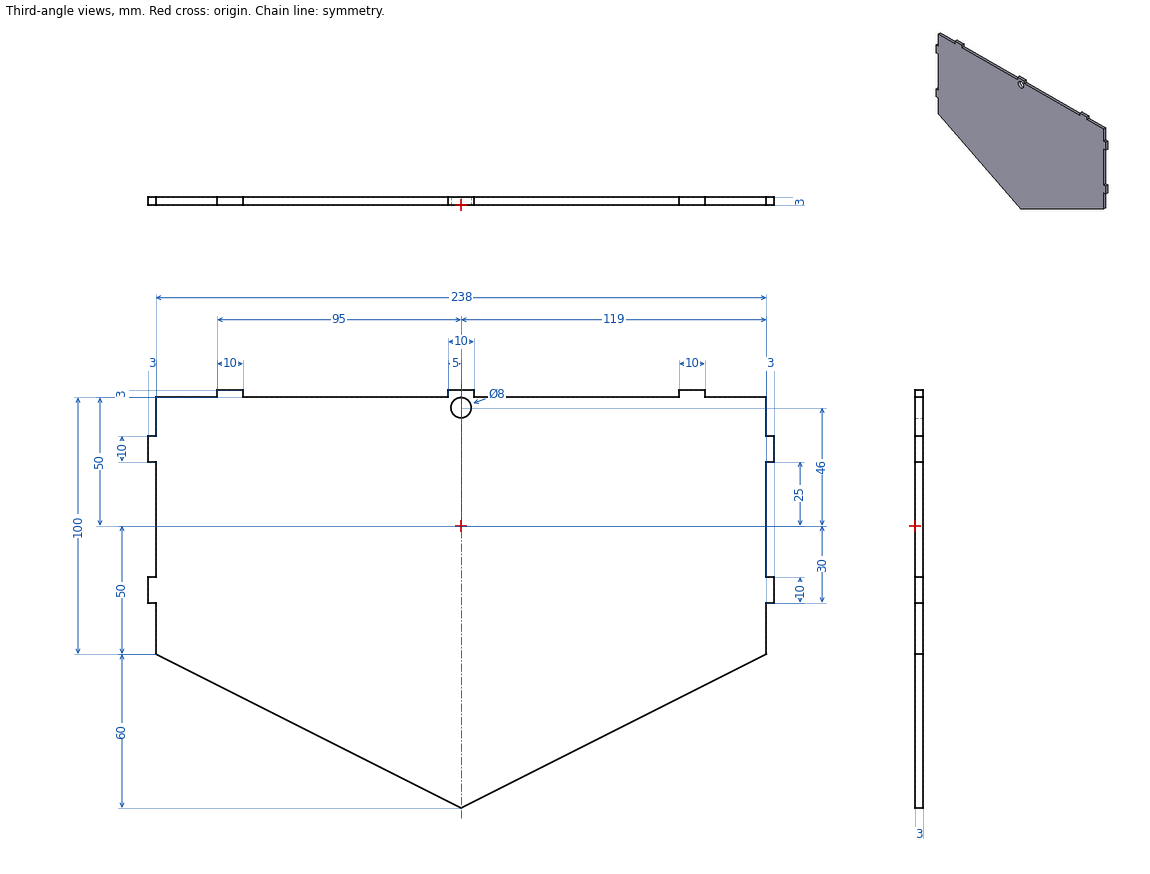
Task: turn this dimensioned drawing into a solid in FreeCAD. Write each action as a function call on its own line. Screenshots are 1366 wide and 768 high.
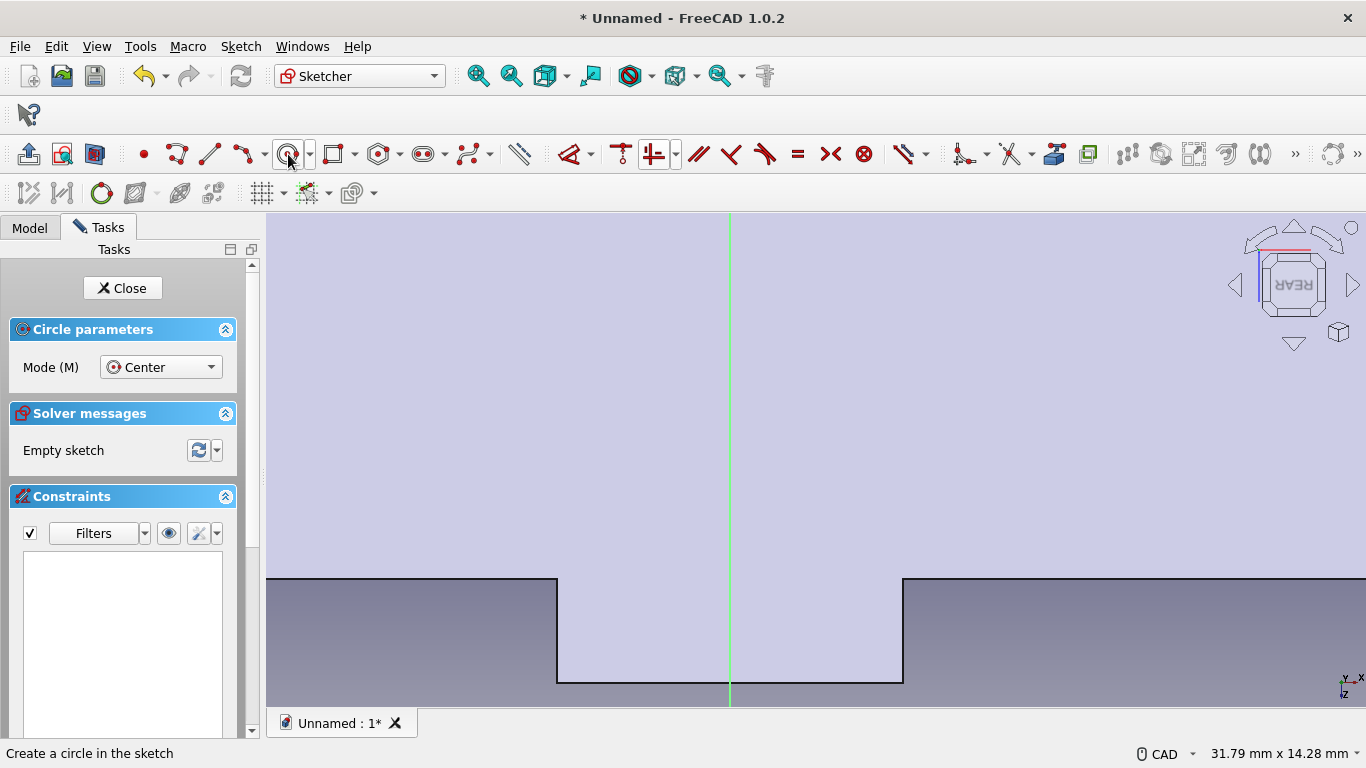
click(730, 441)
move(828, 343)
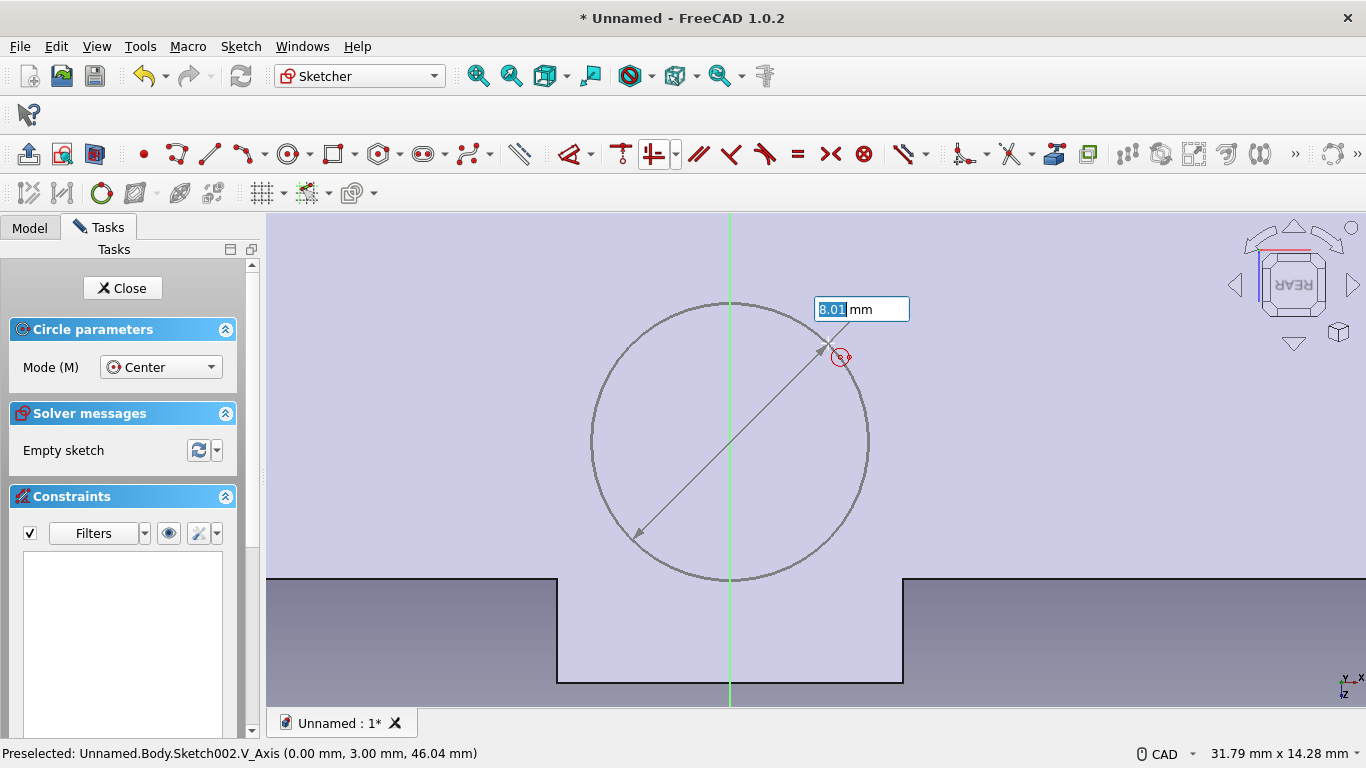
text(8)
key(Return)
key(Escape)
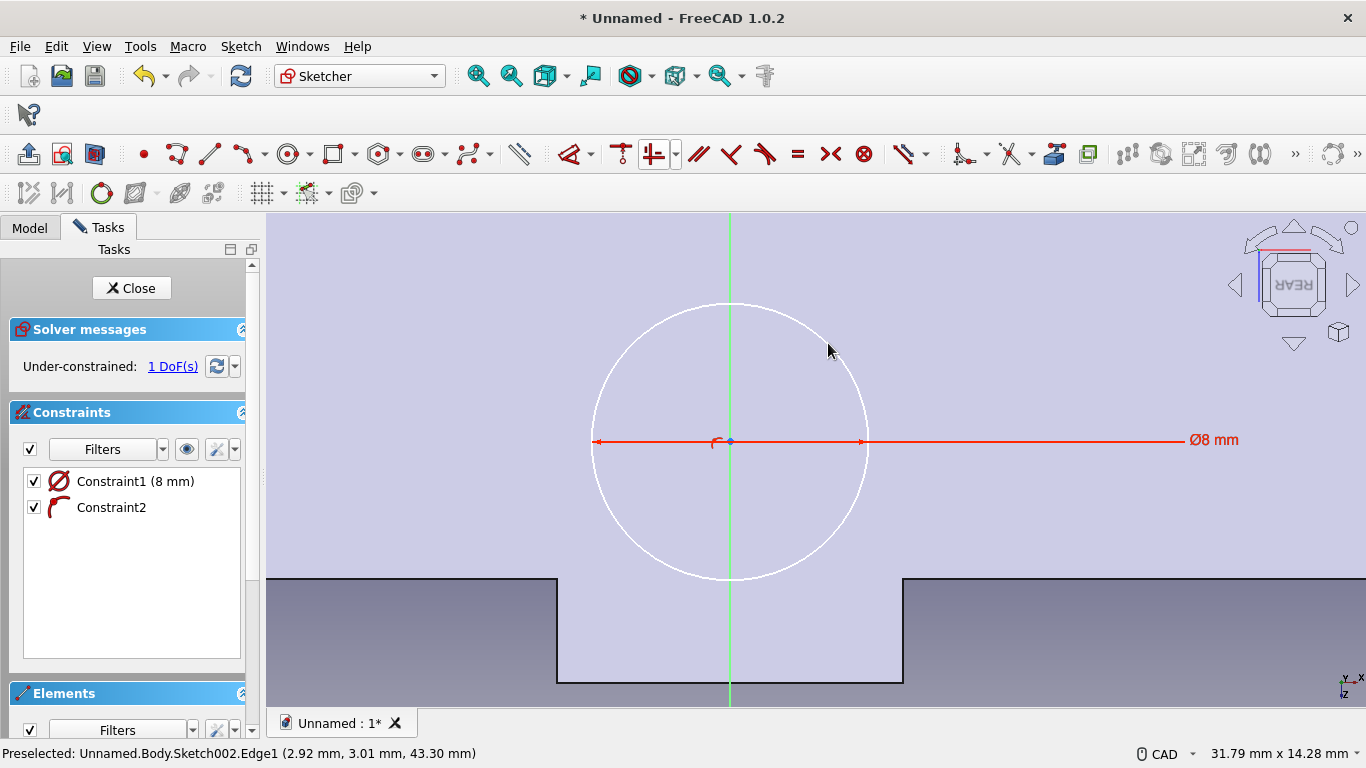
click(568, 154)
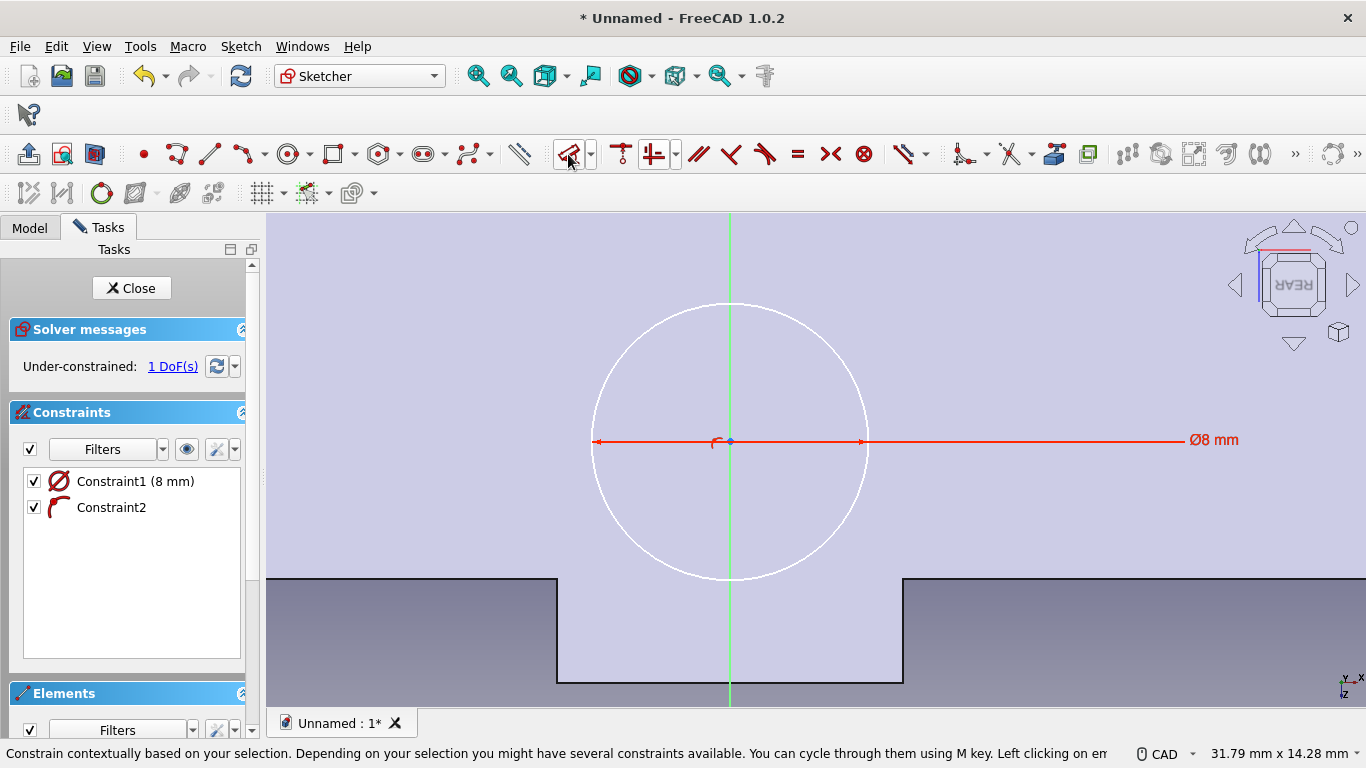
click(730, 442)
click(764, 341)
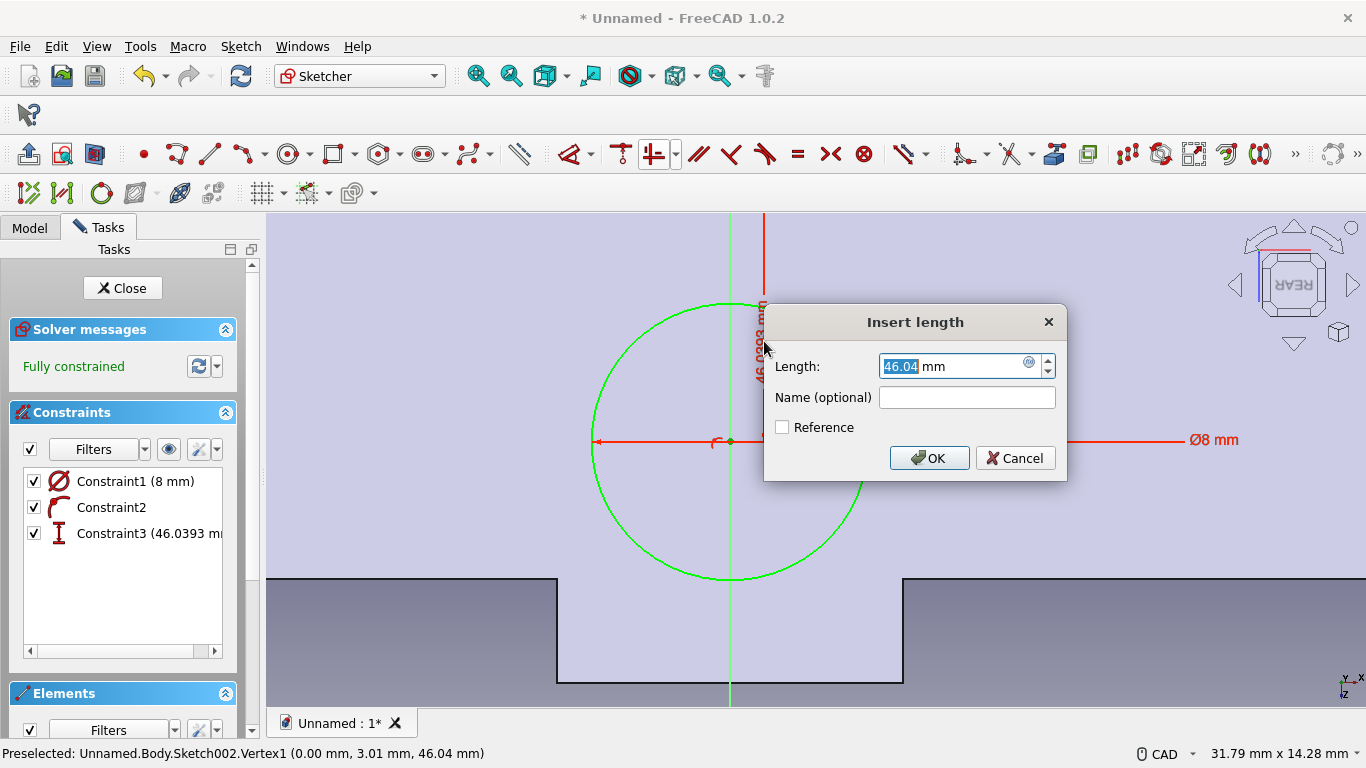
text(46)
key(Return)
key(Escape)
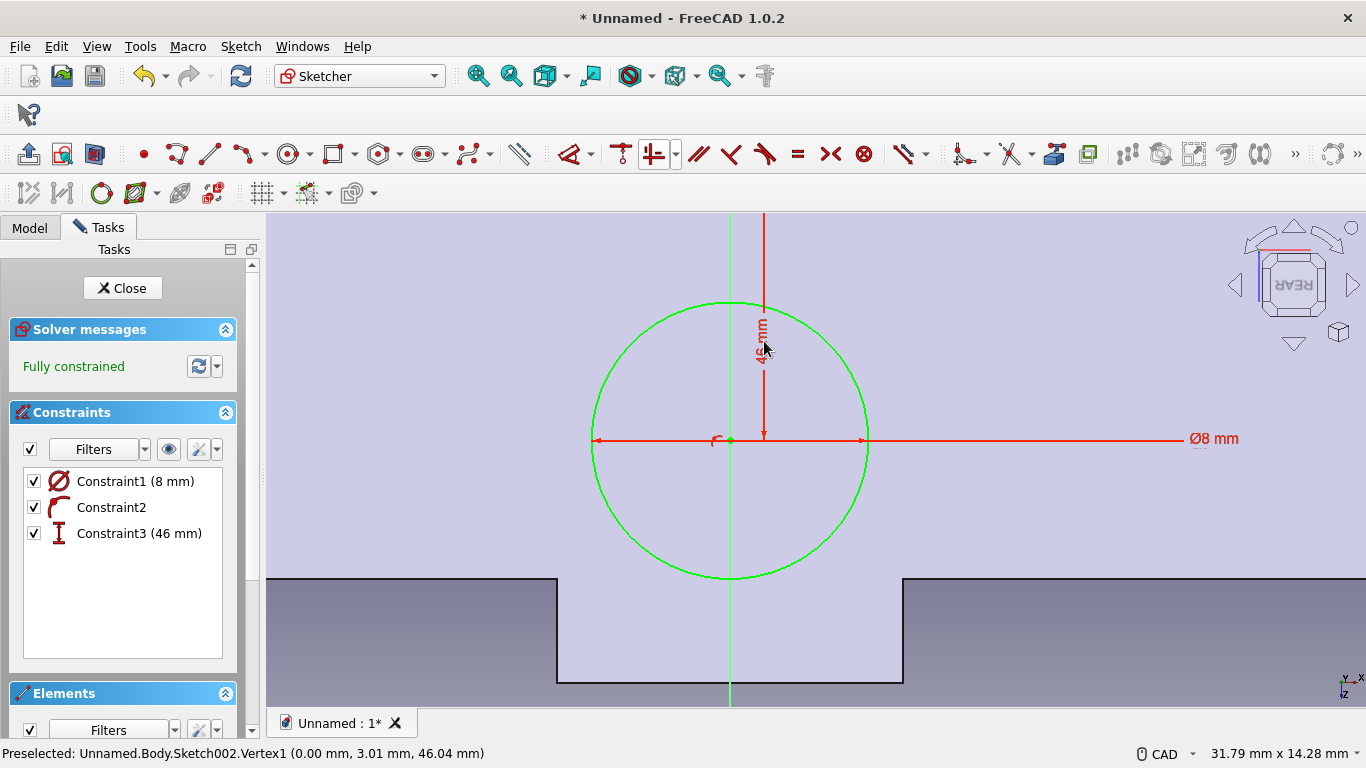
click(123, 288)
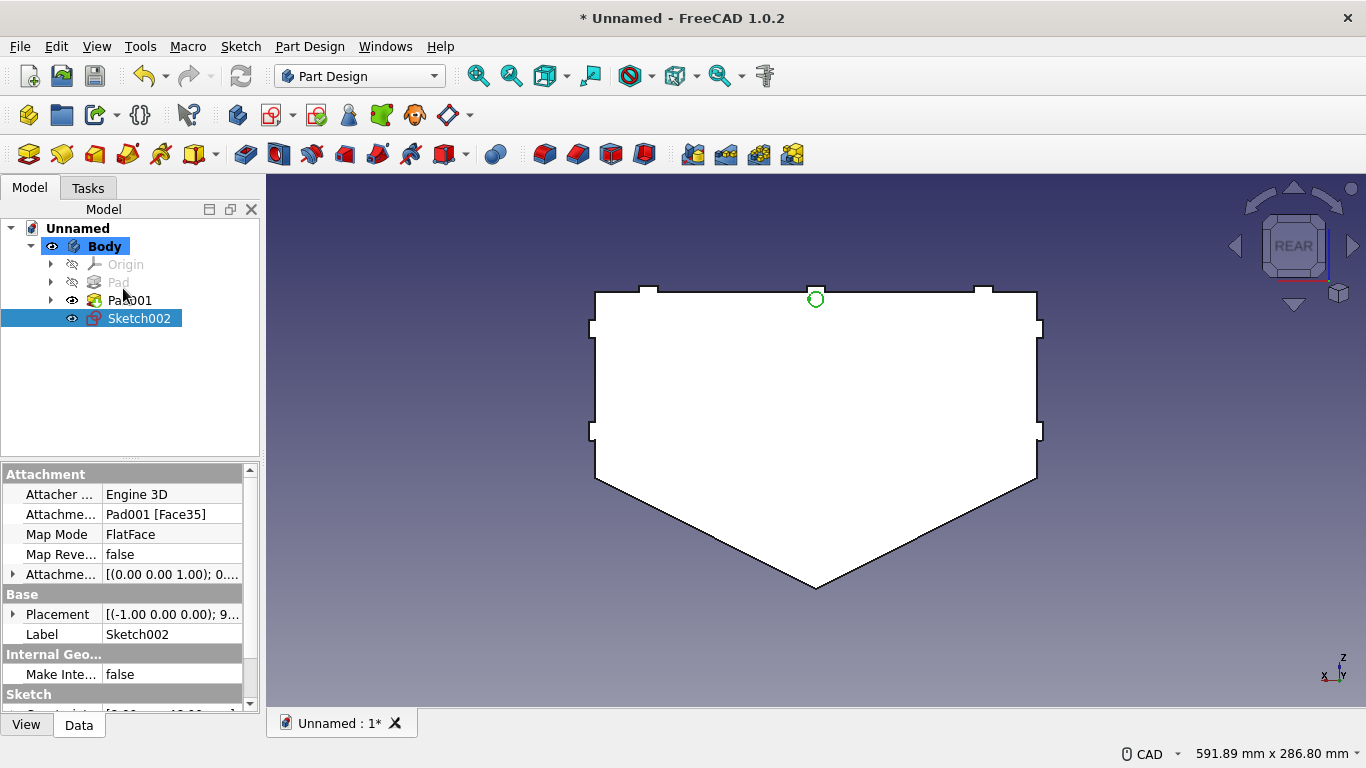
click(246, 154)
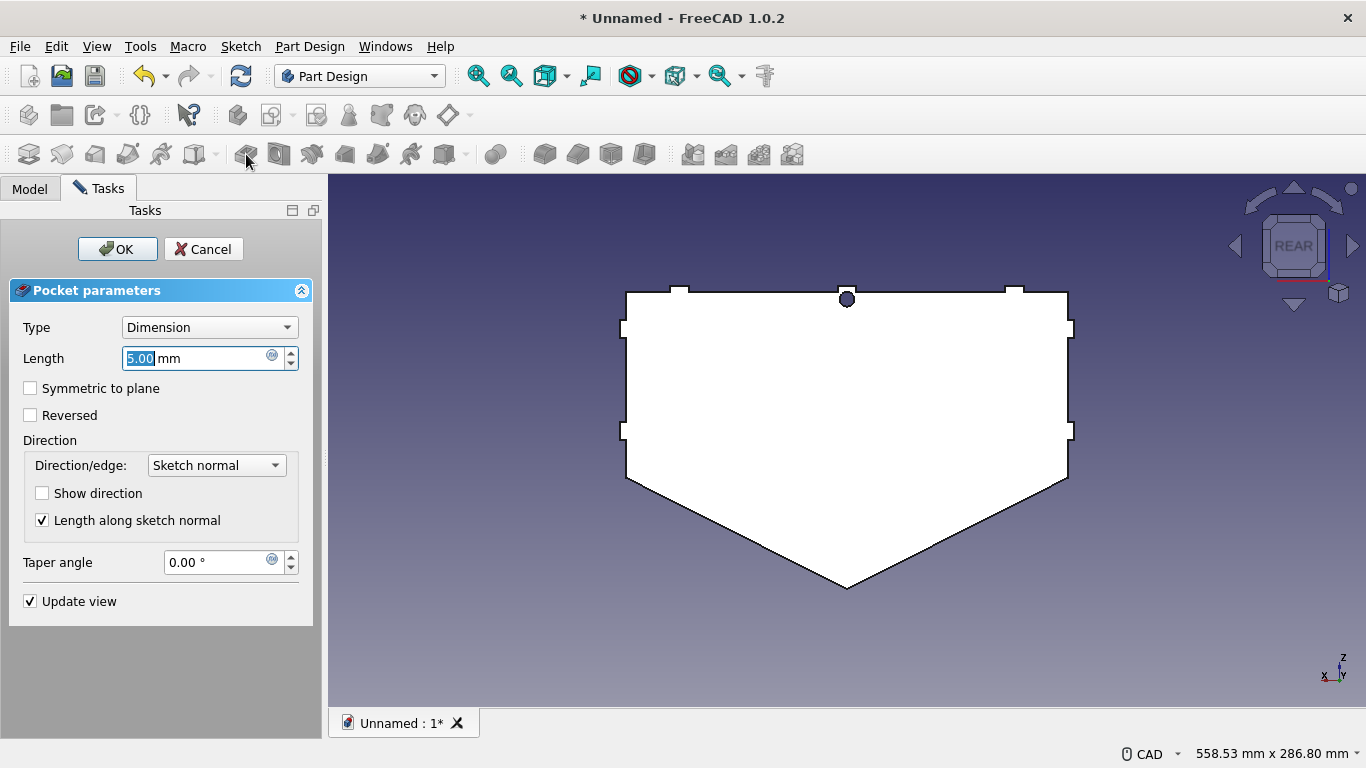
click(210, 328)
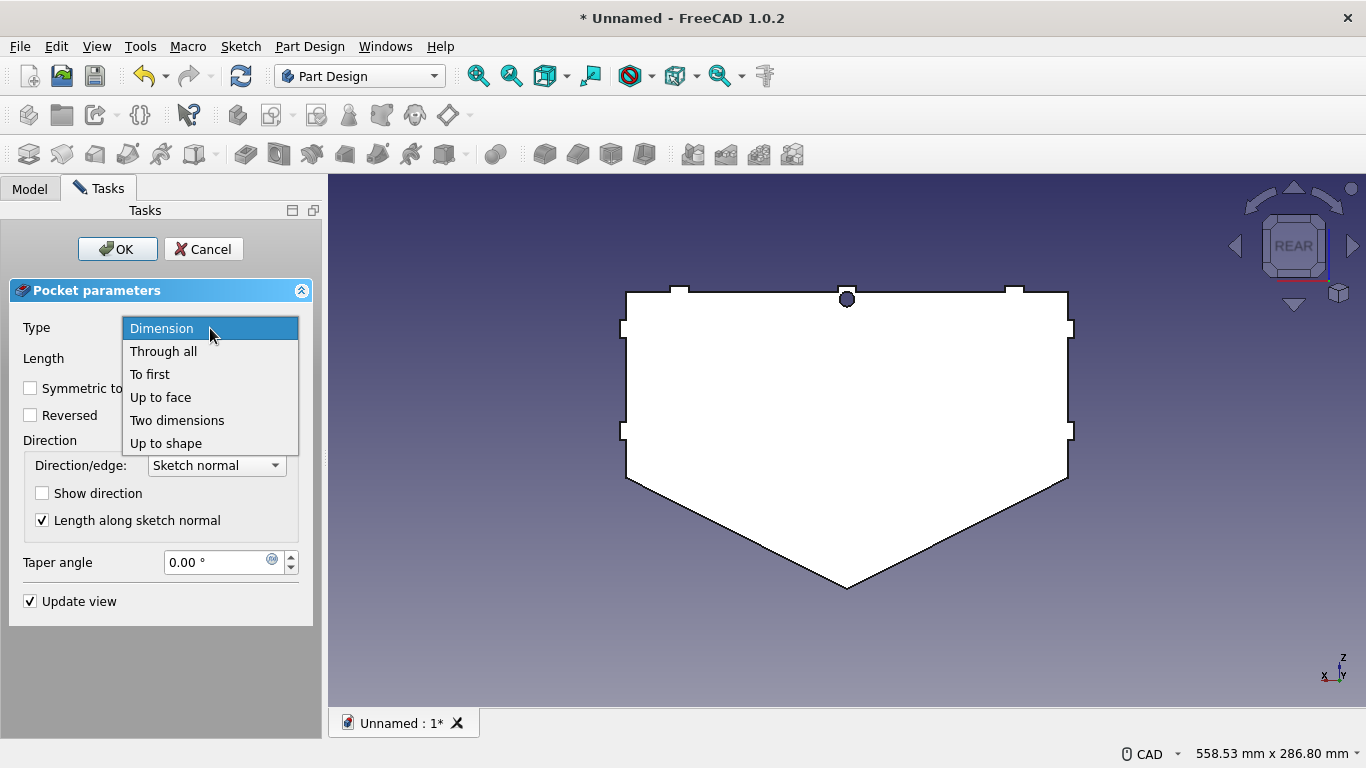
click(208, 352)